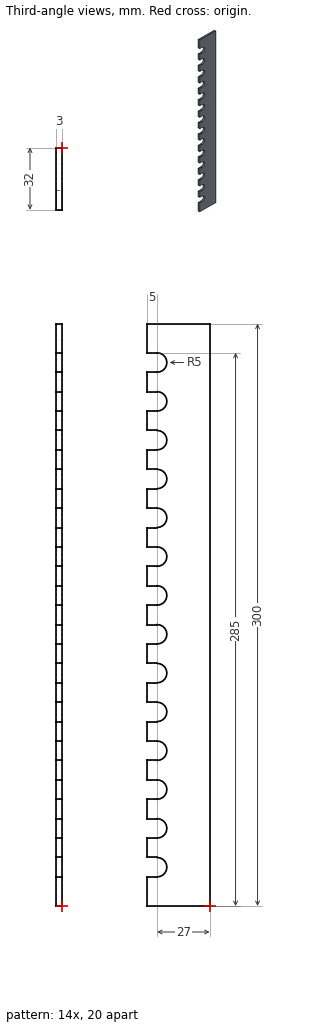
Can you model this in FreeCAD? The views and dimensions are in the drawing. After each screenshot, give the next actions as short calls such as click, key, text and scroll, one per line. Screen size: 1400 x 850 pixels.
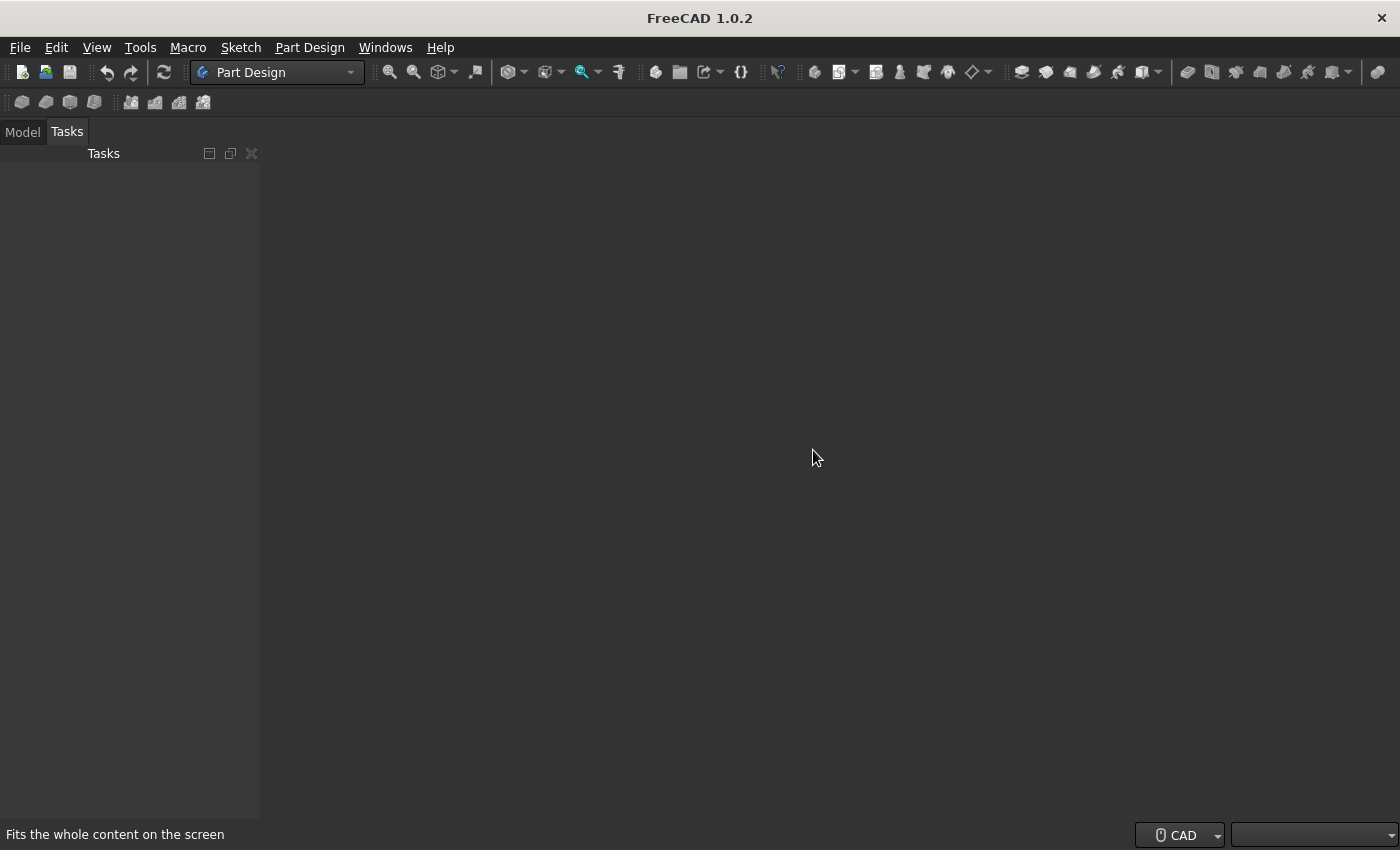
click(22, 72)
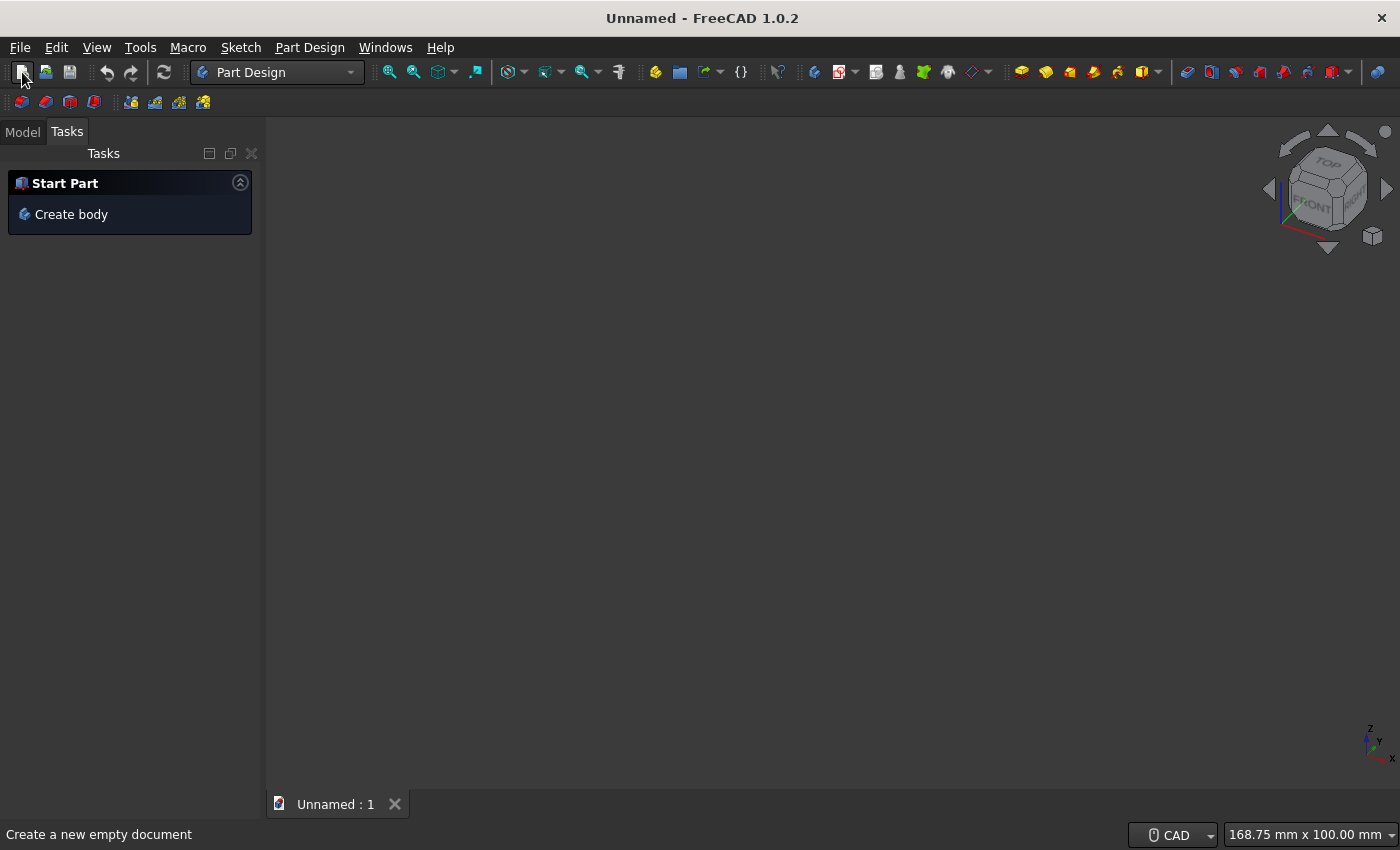
click(840, 72)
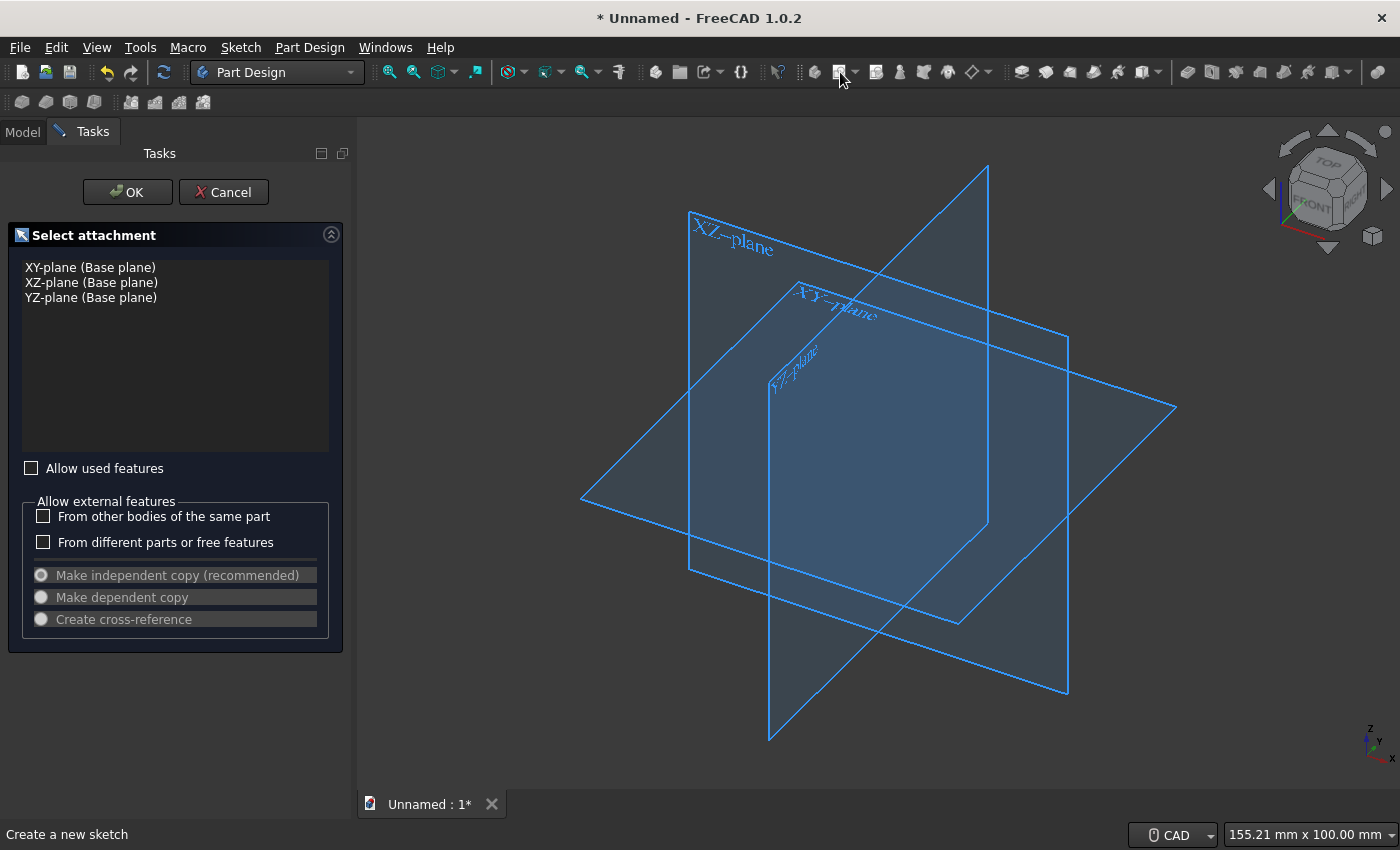
click(82, 268)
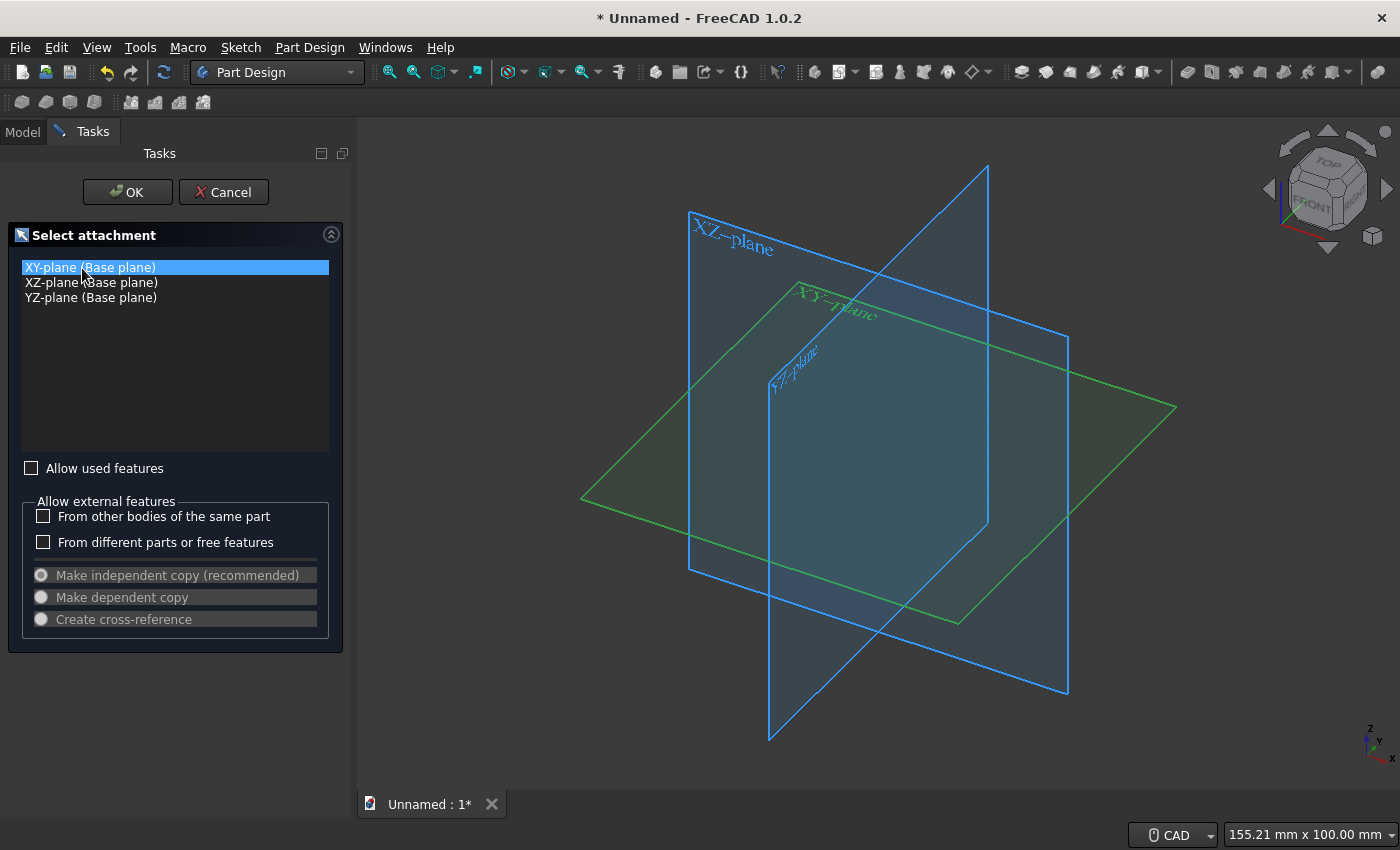
click(128, 192)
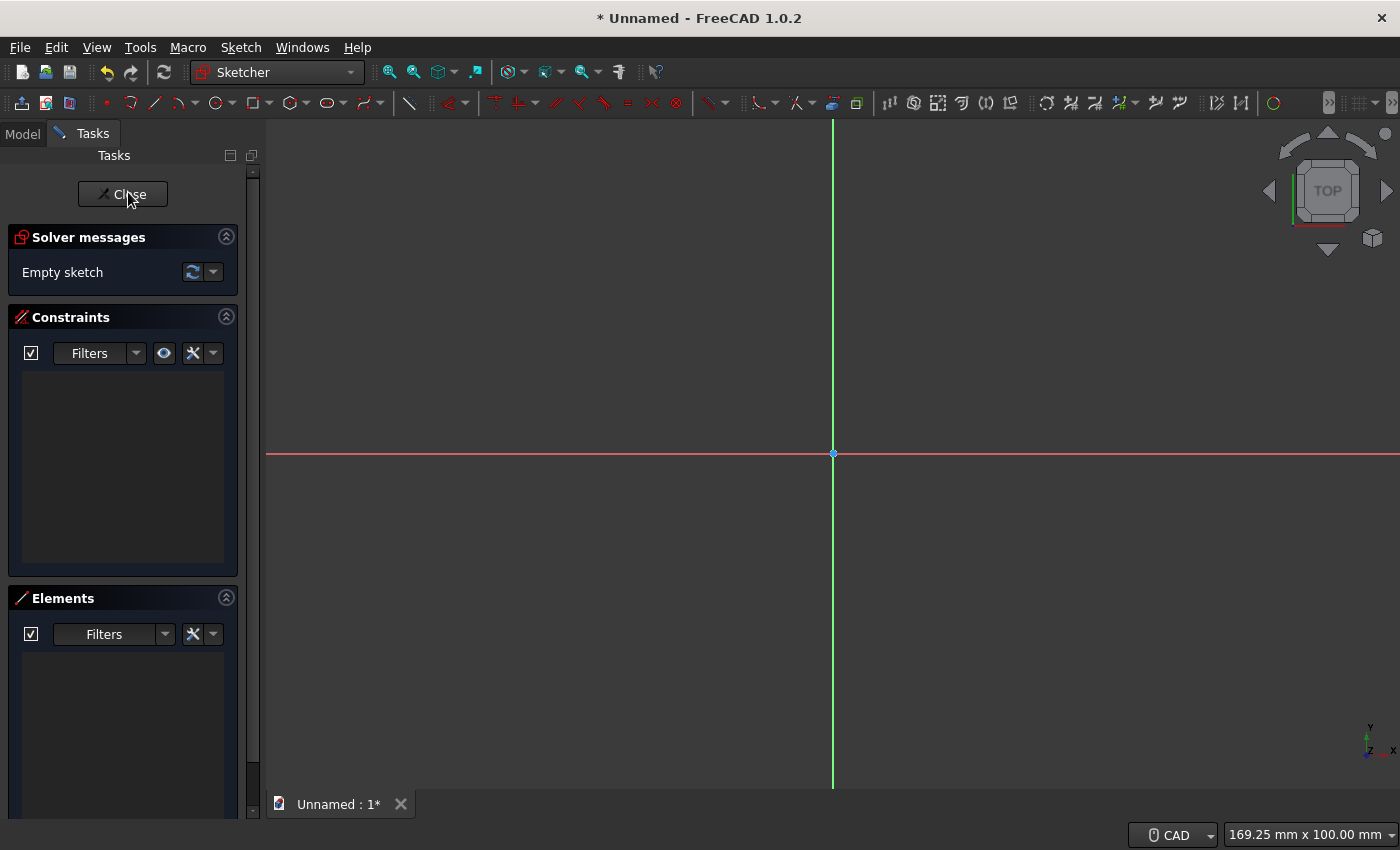
scroll(871, 649, up, 4)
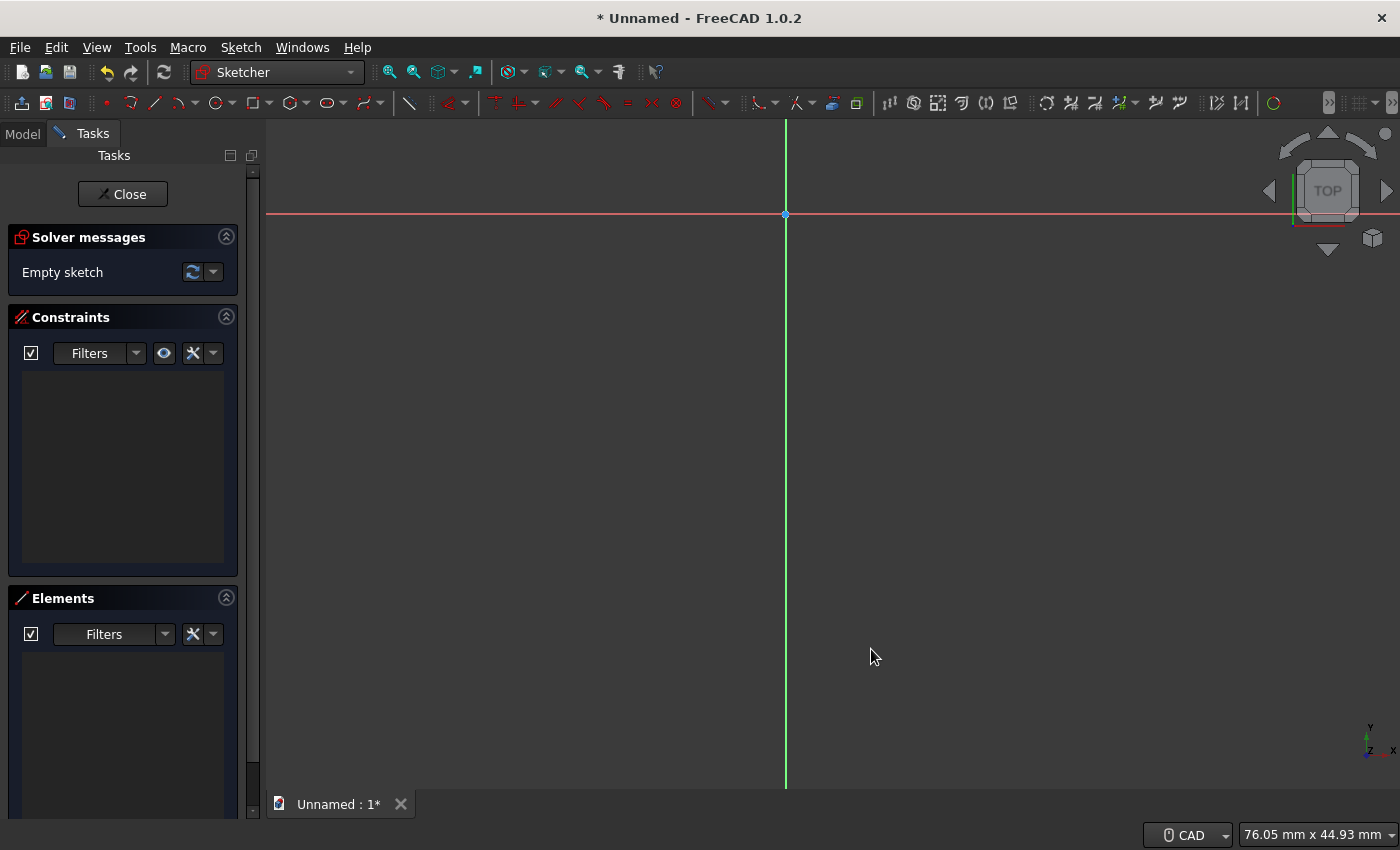
key(g)
key(r)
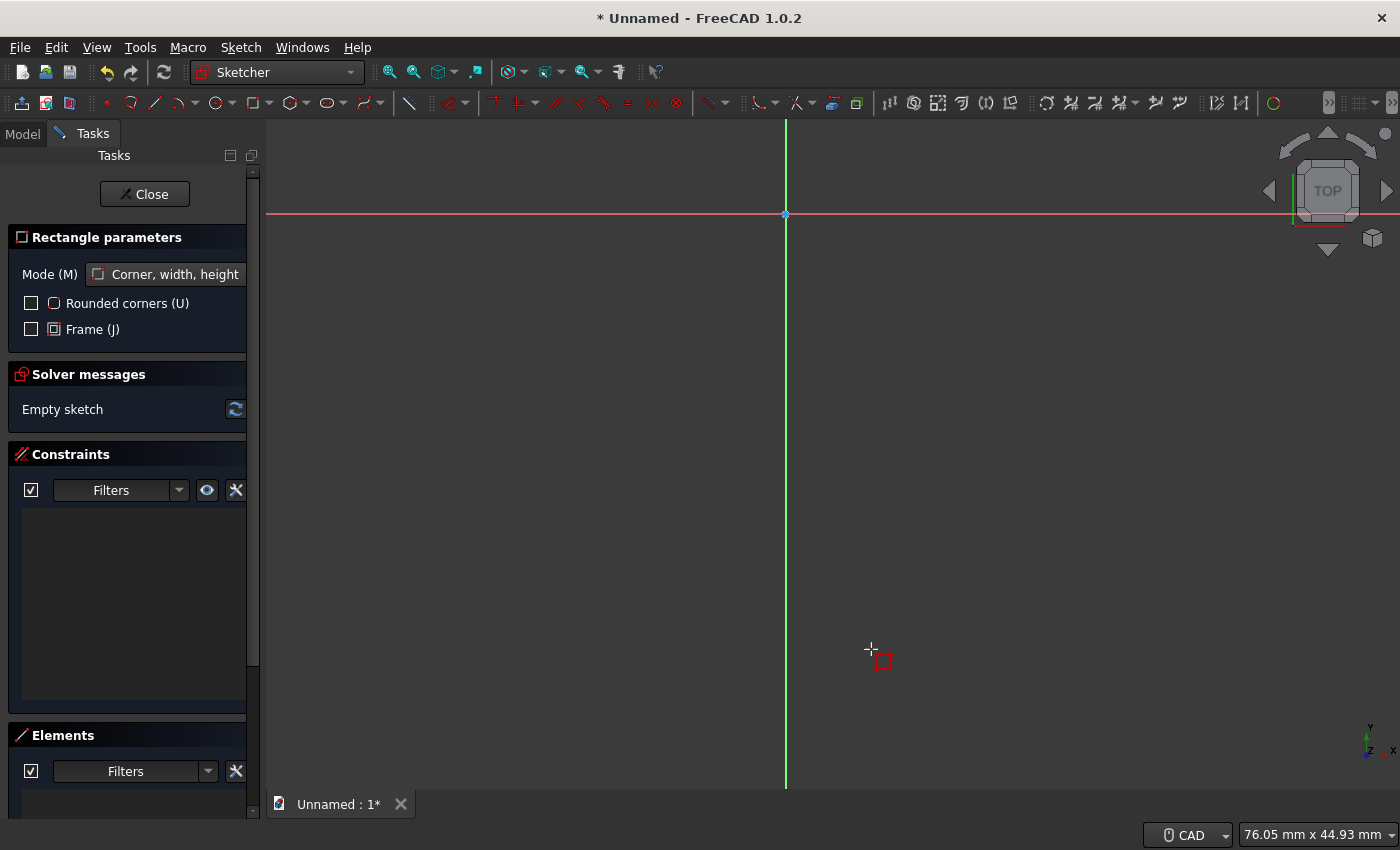
click(786, 214)
click(741, 691)
key(Escape)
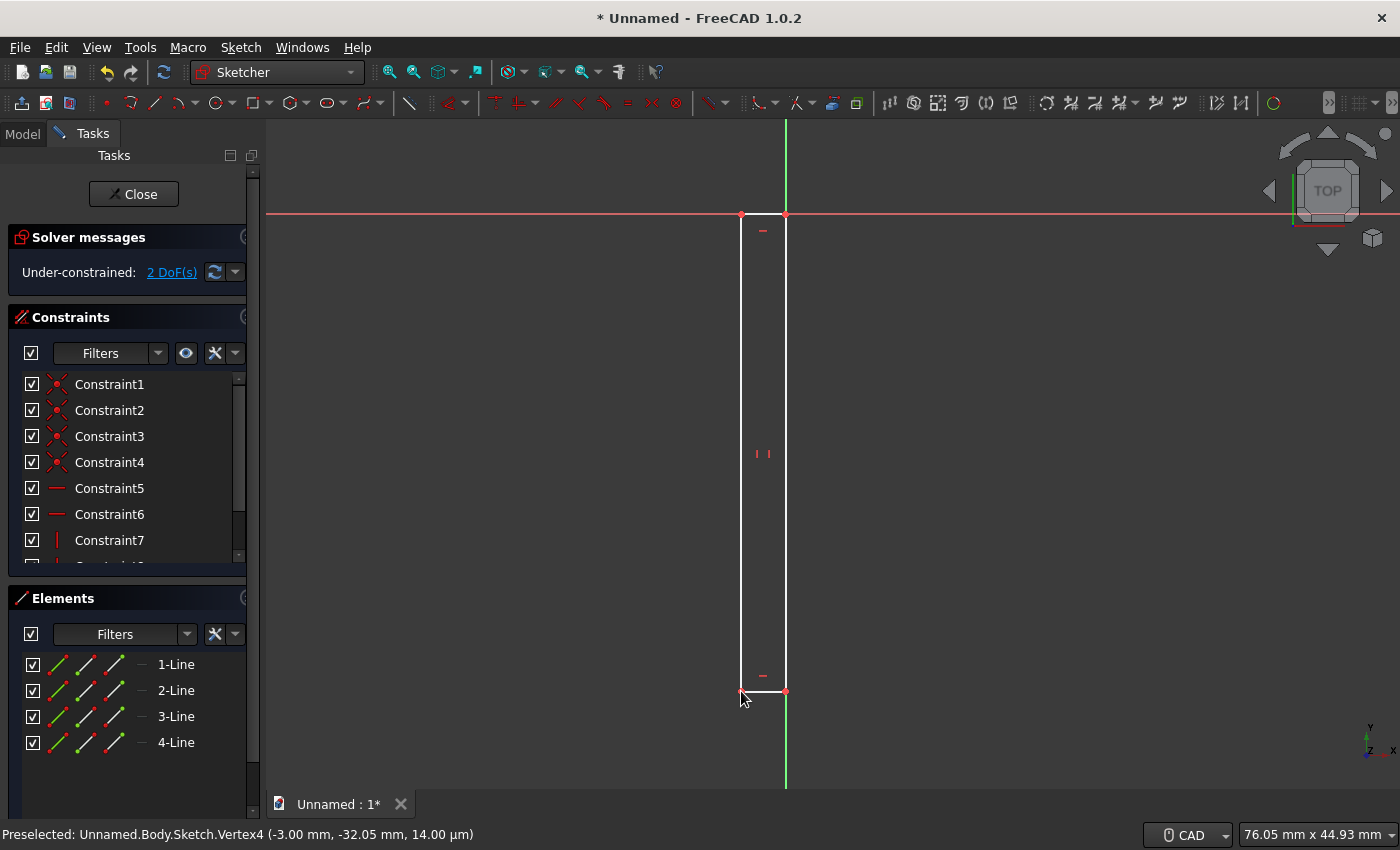
click(448, 104)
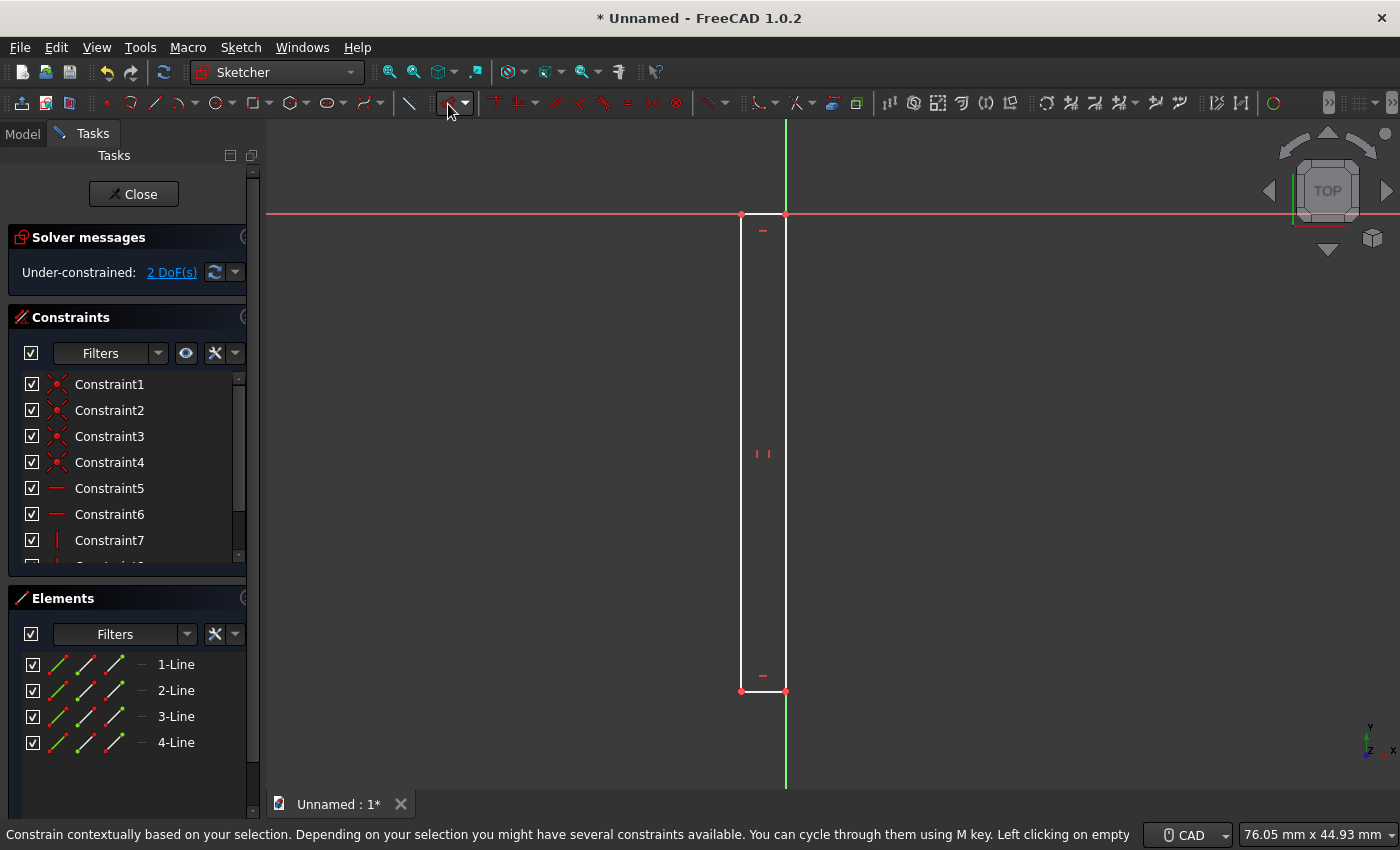
click(772, 214)
click(763, 180)